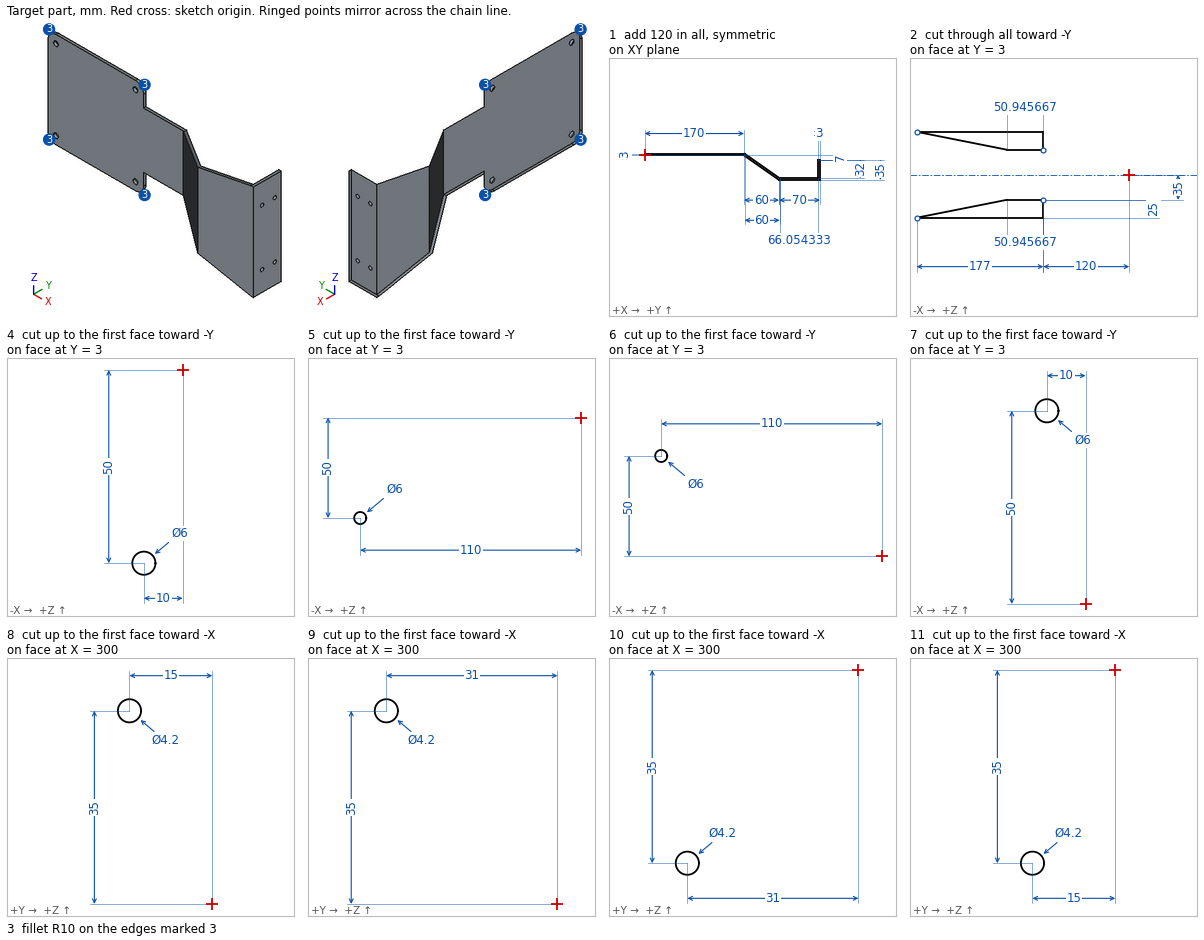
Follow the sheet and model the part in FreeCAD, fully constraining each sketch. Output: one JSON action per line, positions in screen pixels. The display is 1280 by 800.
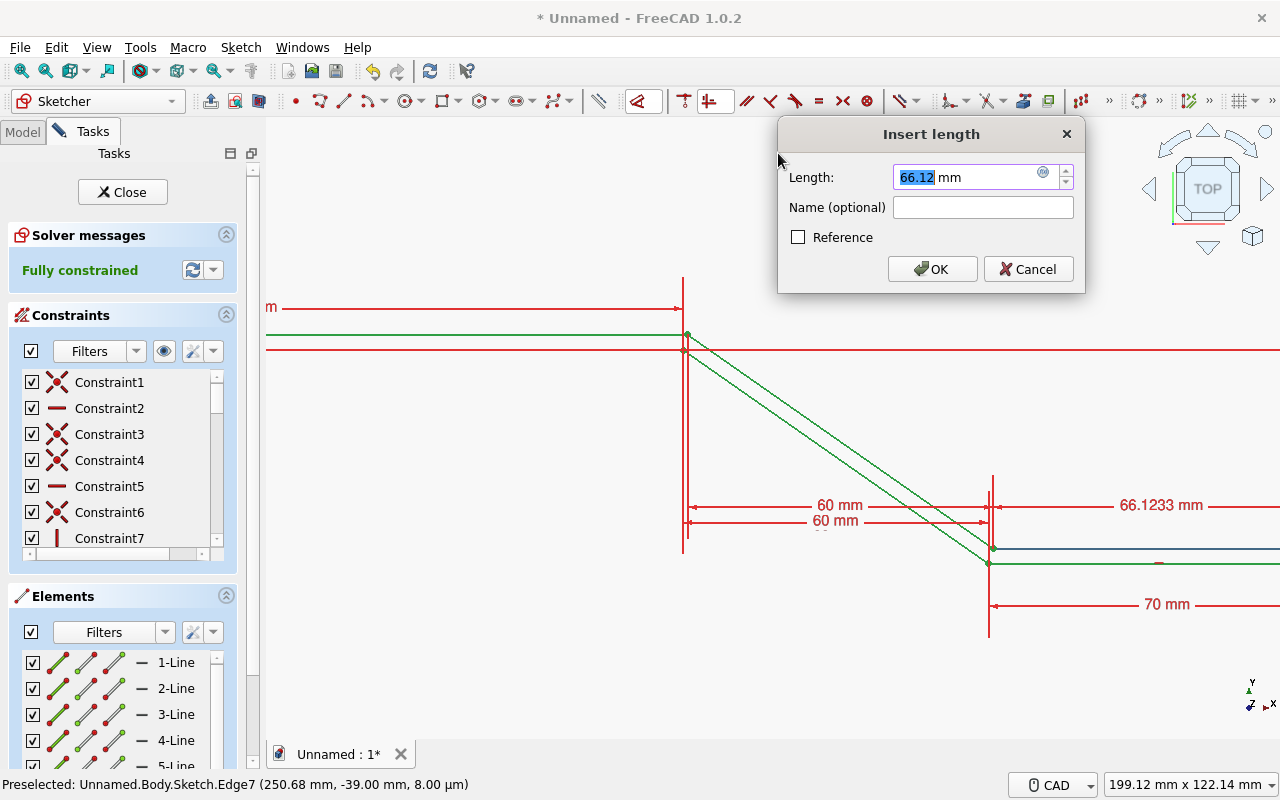
{"action": "type", "text": "66.054333"}
{"action": "key", "text": "Return"}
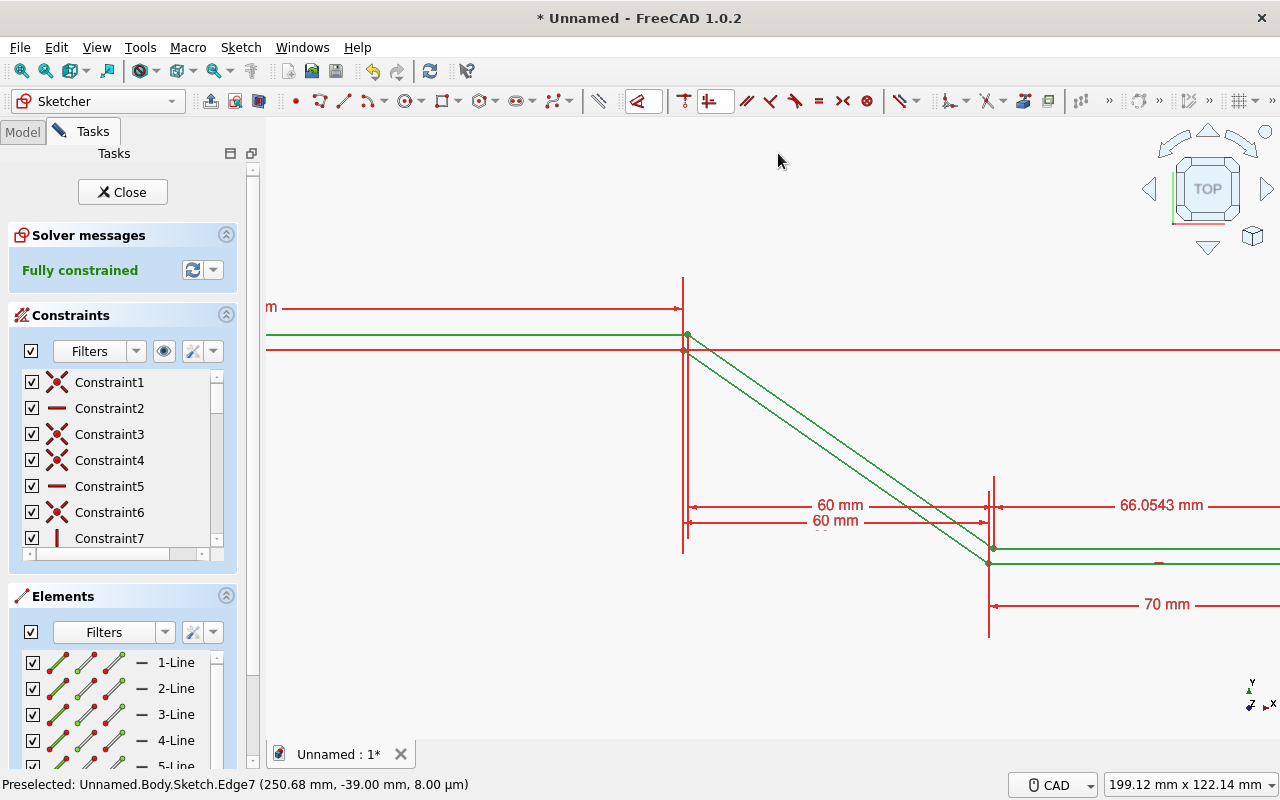
{"action": "left_click", "coordinate": [123, 192]}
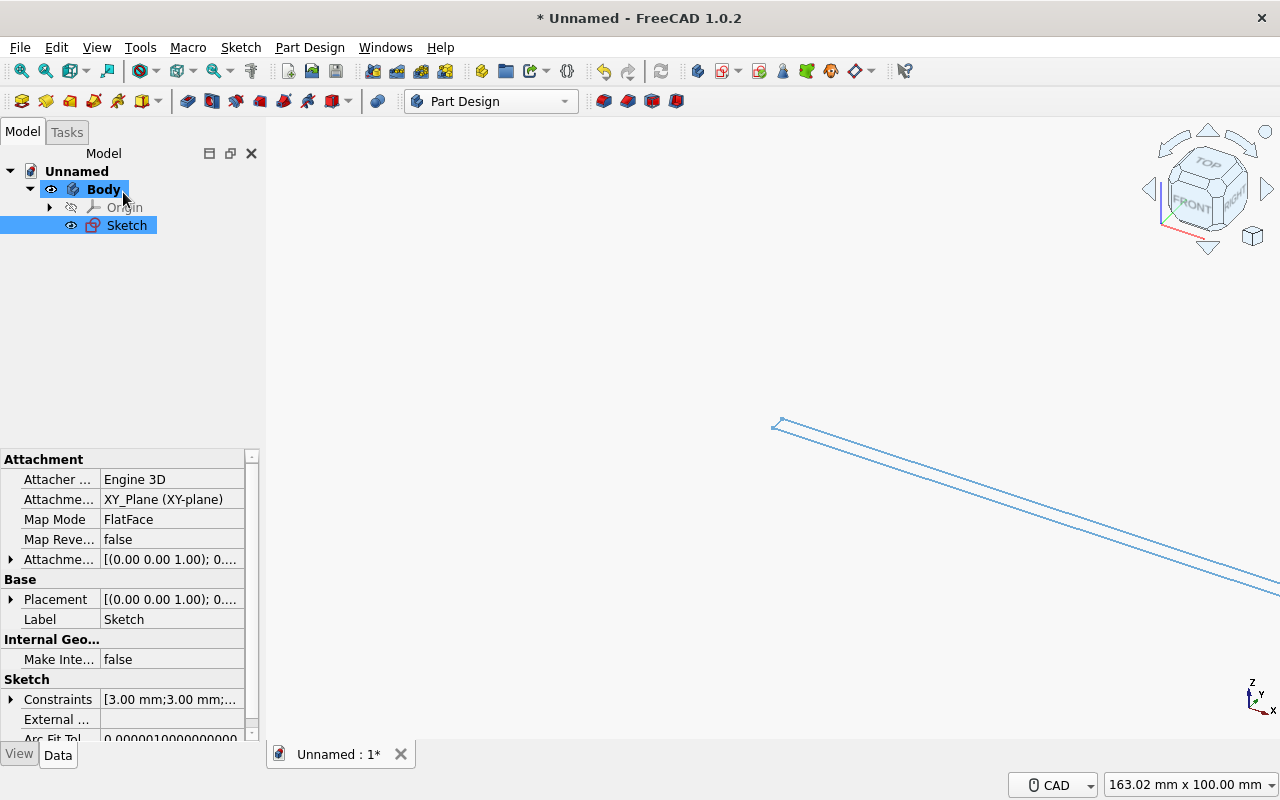
{"action": "left_click", "coordinate": [22, 102]}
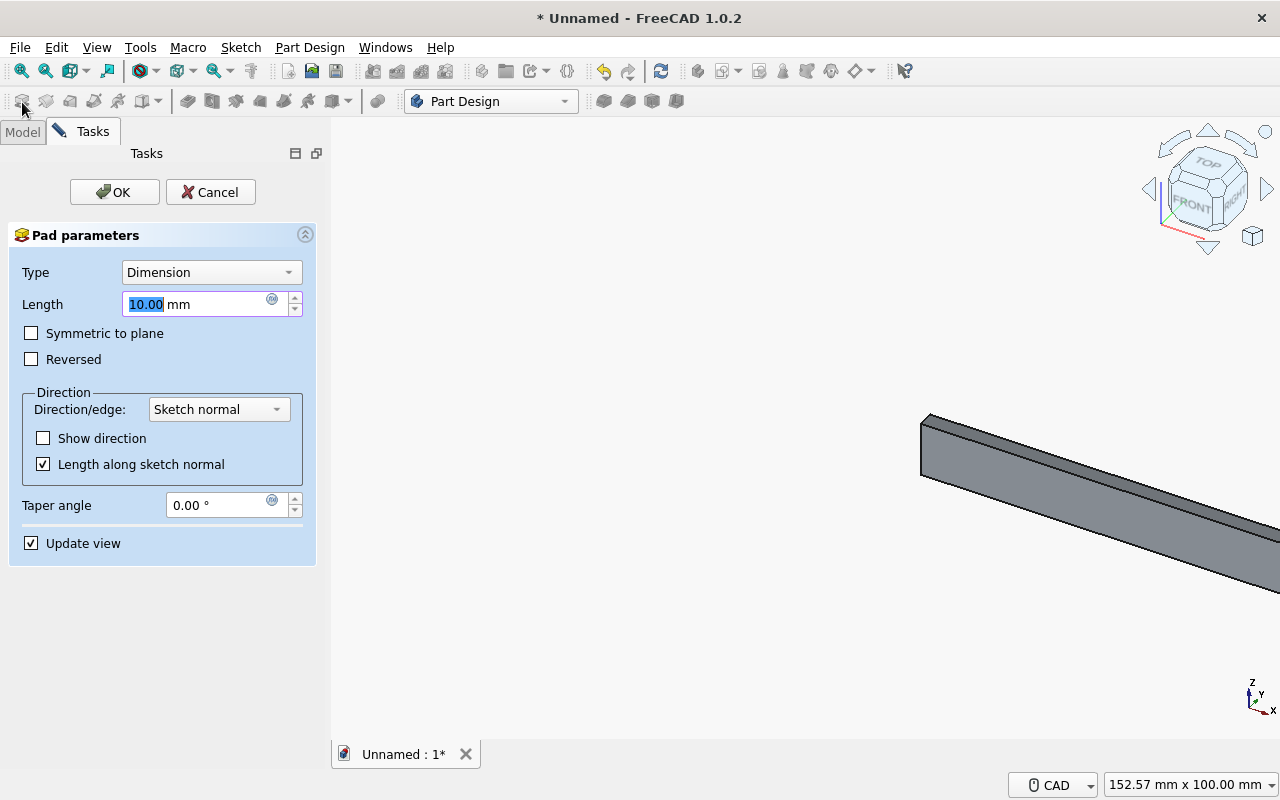
{"action": "type", "text": "120"}
{"action": "key", "text": "Tab"}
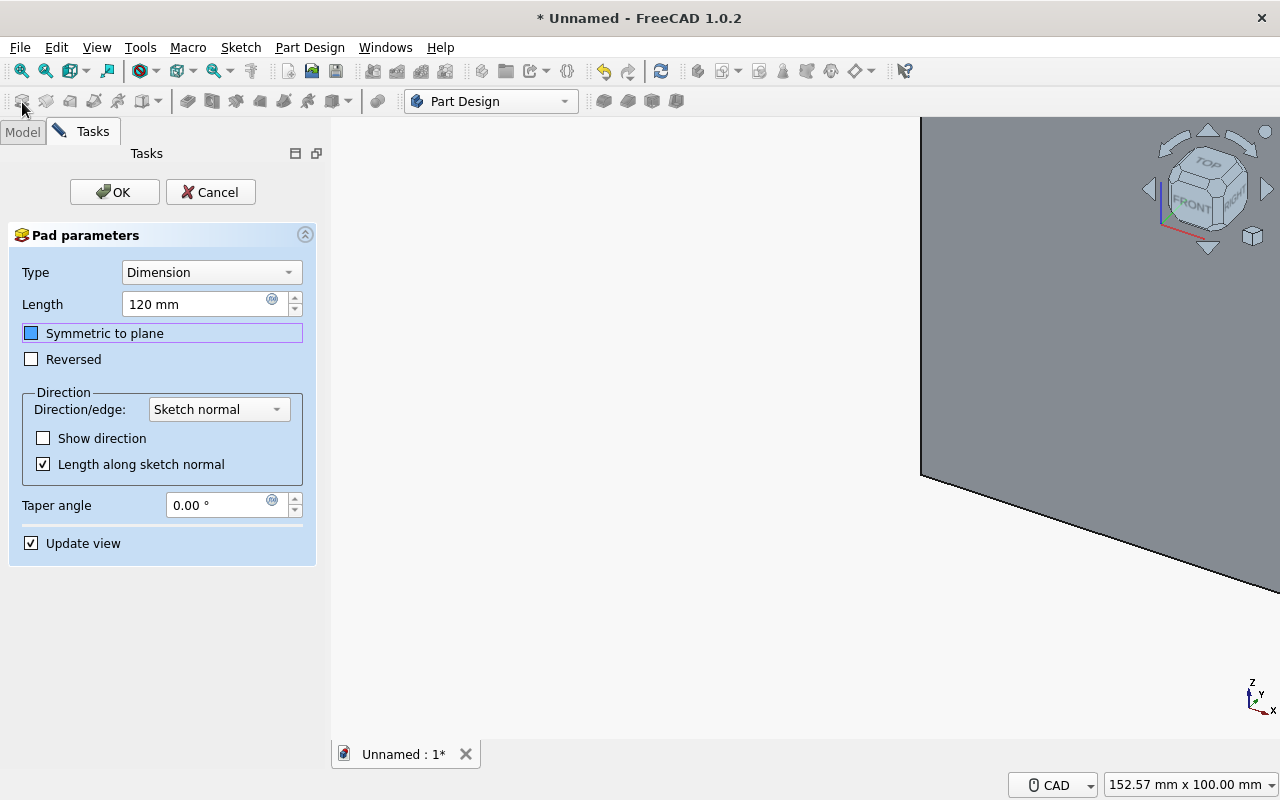
{"action": "left_click", "coordinate": [30, 333]}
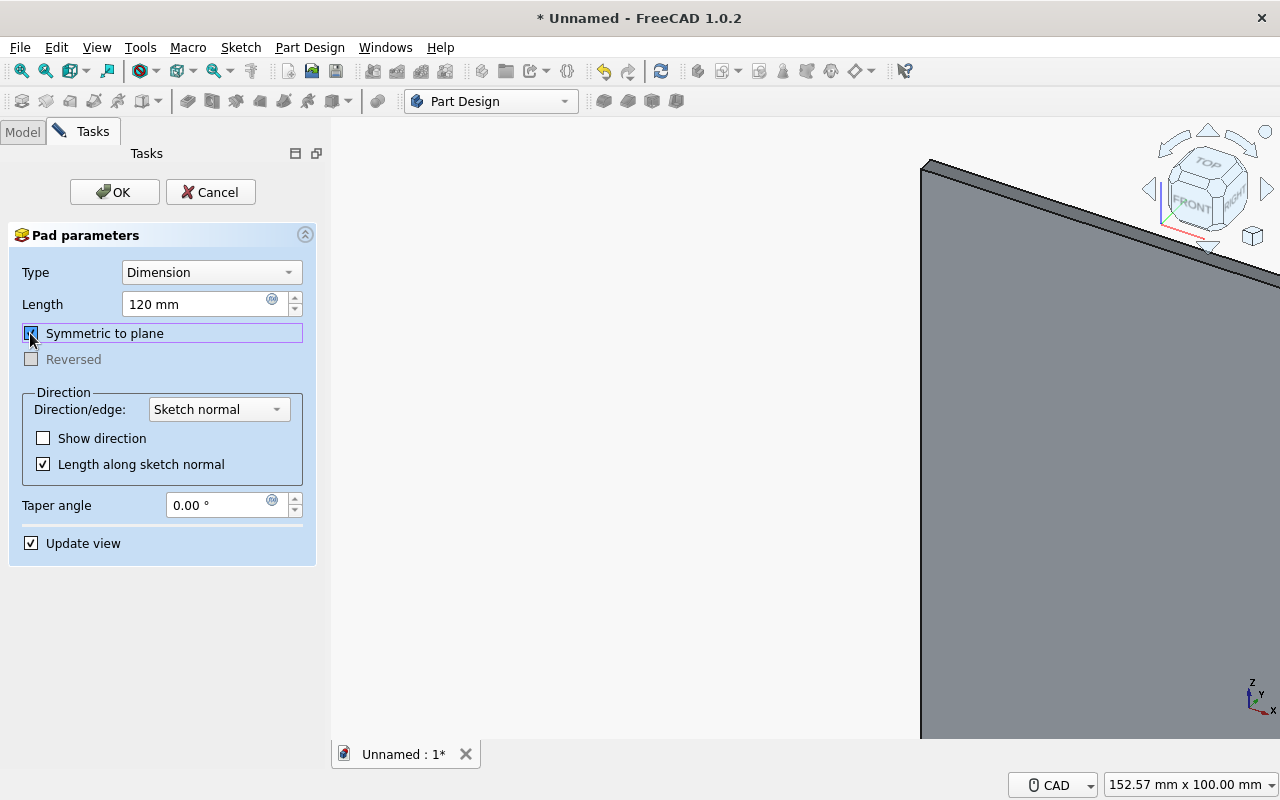
{"action": "left_click", "coordinate": [115, 192]}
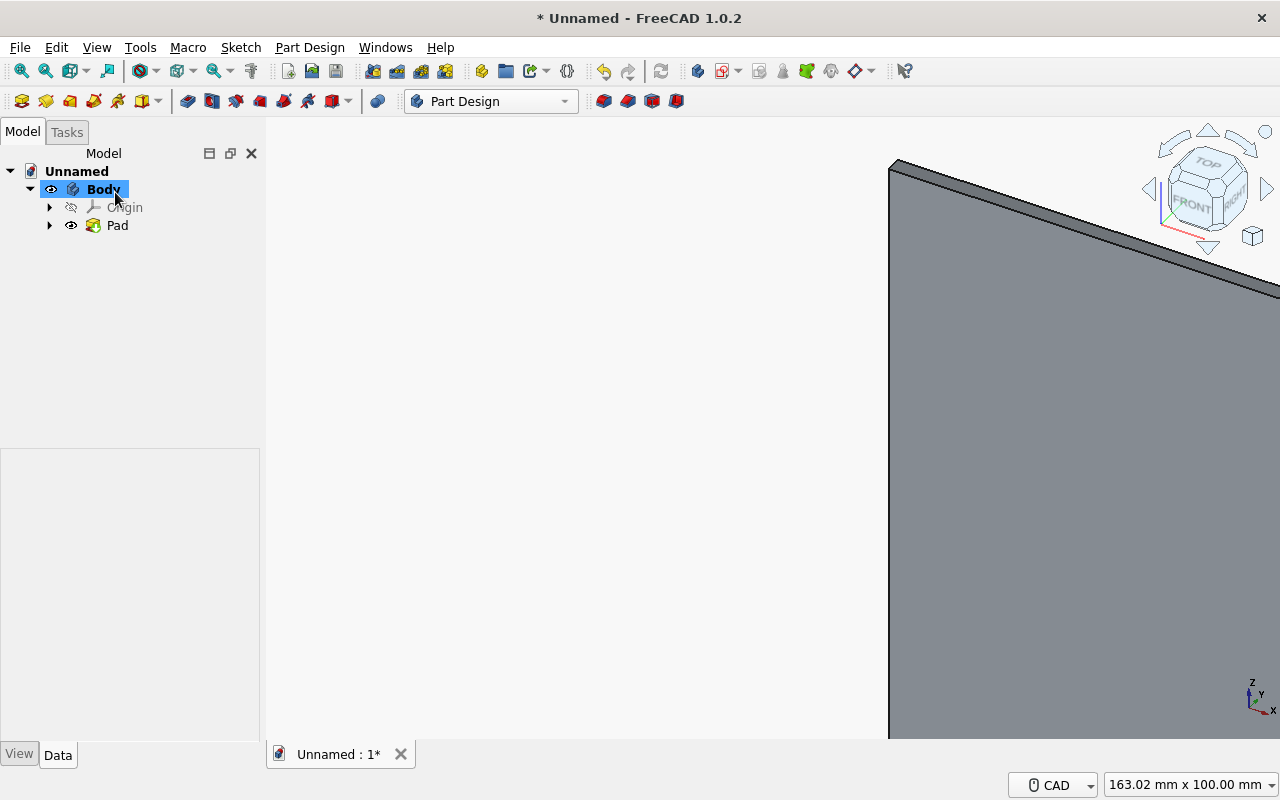
{"action": "left_click", "coordinate": [22, 72]}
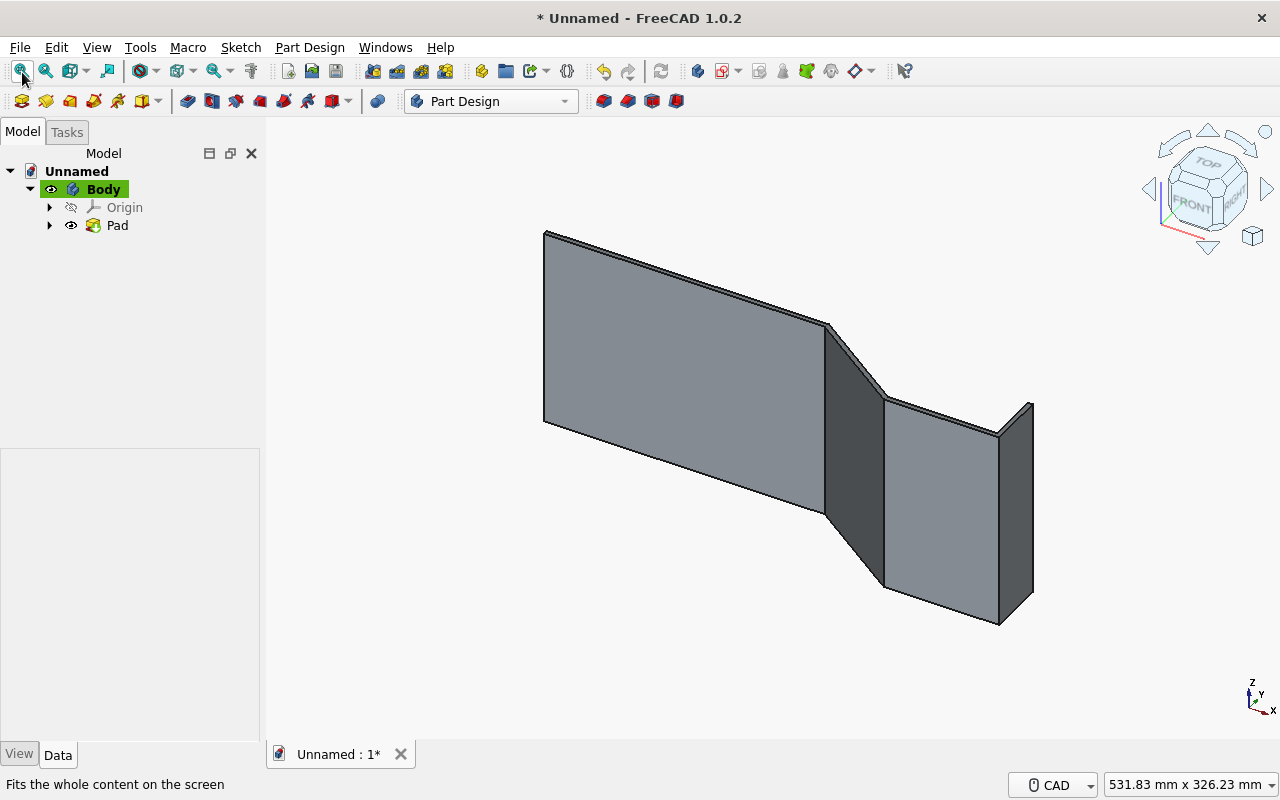
{"action": "key", "text": "4"}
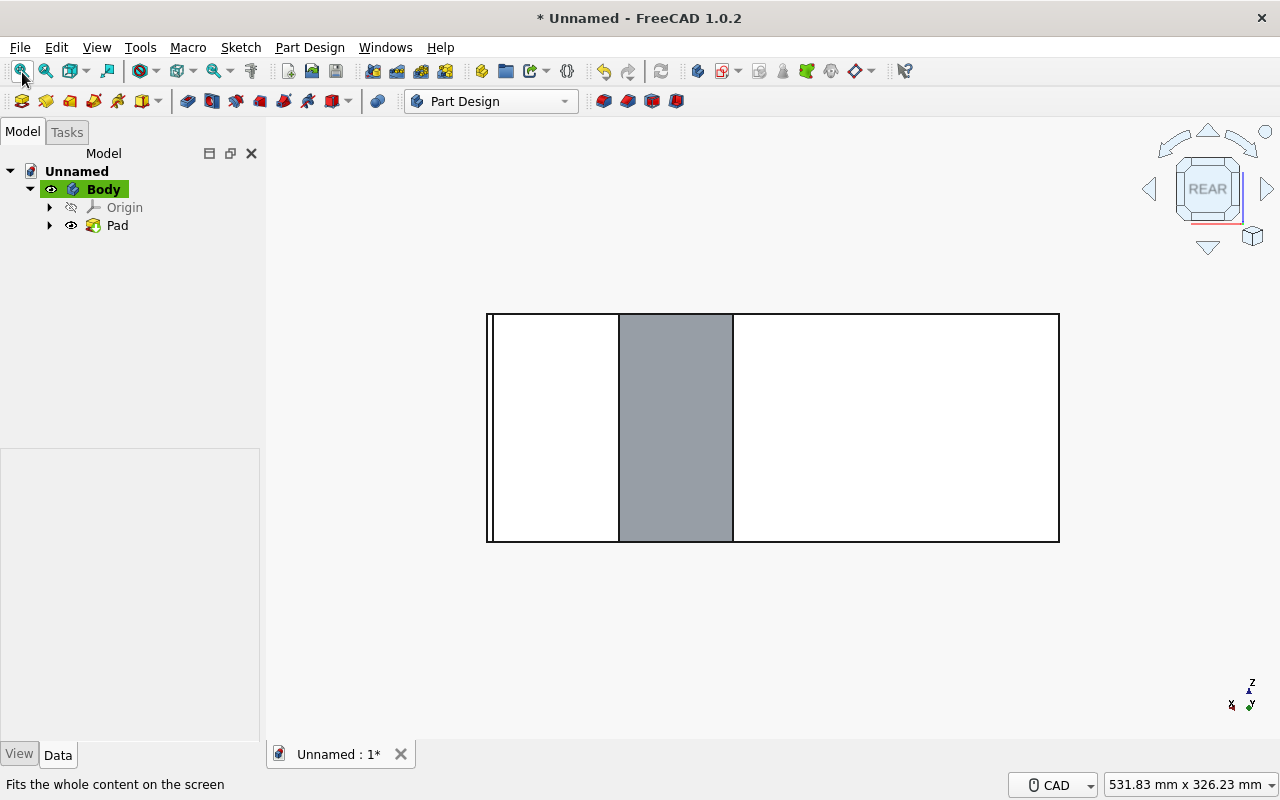
{"action": "left_click", "coordinate": [849, 427]}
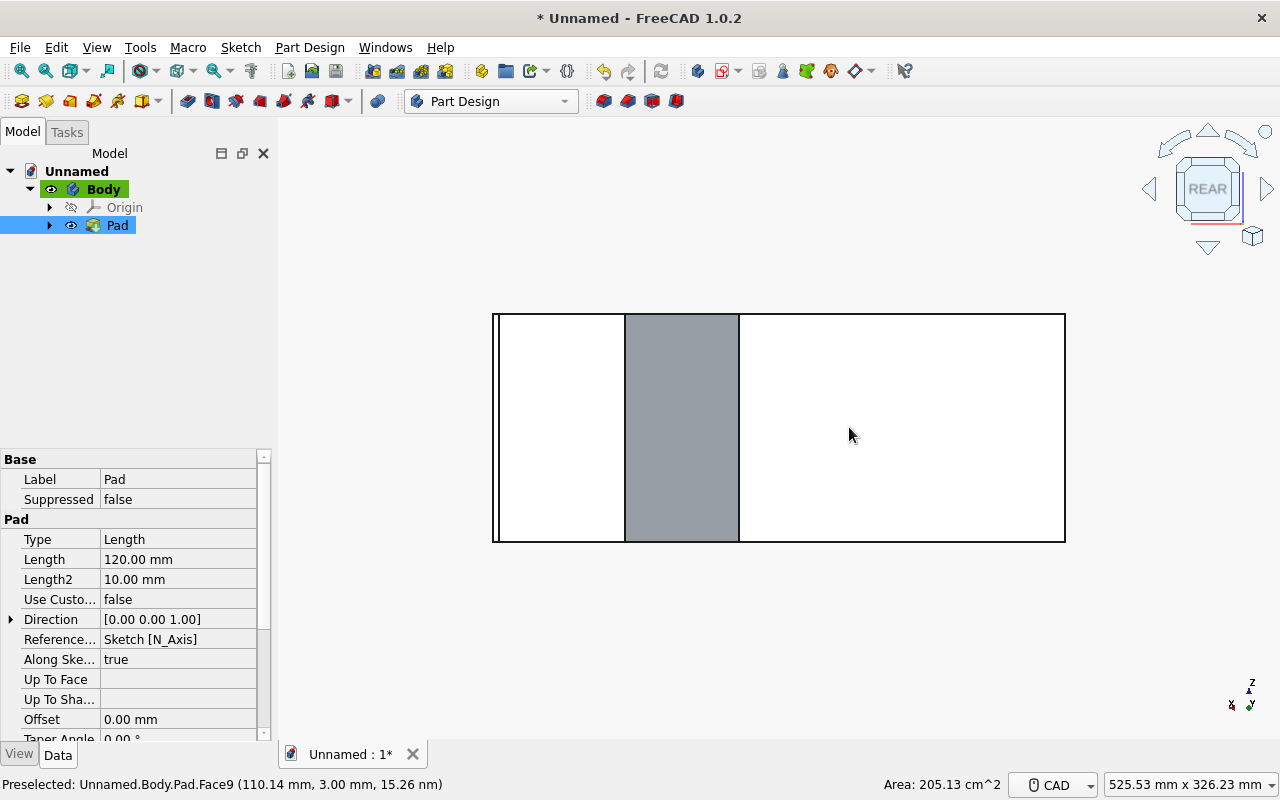
{"action": "left_click", "coordinate": [722, 72]}